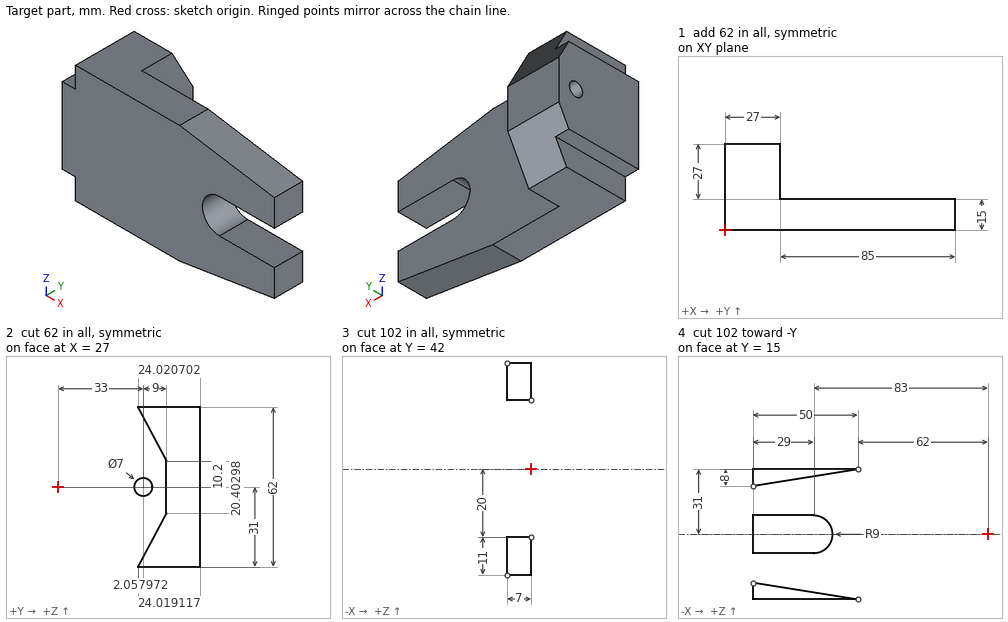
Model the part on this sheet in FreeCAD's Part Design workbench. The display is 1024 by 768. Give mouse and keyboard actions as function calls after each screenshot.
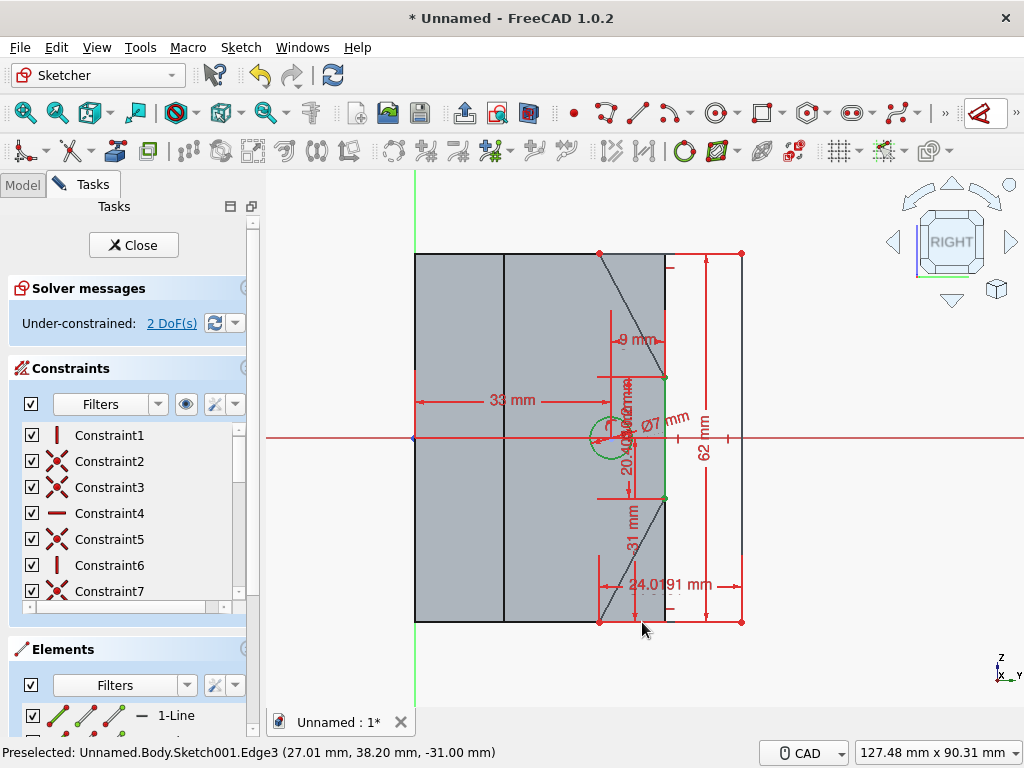
click(699, 254)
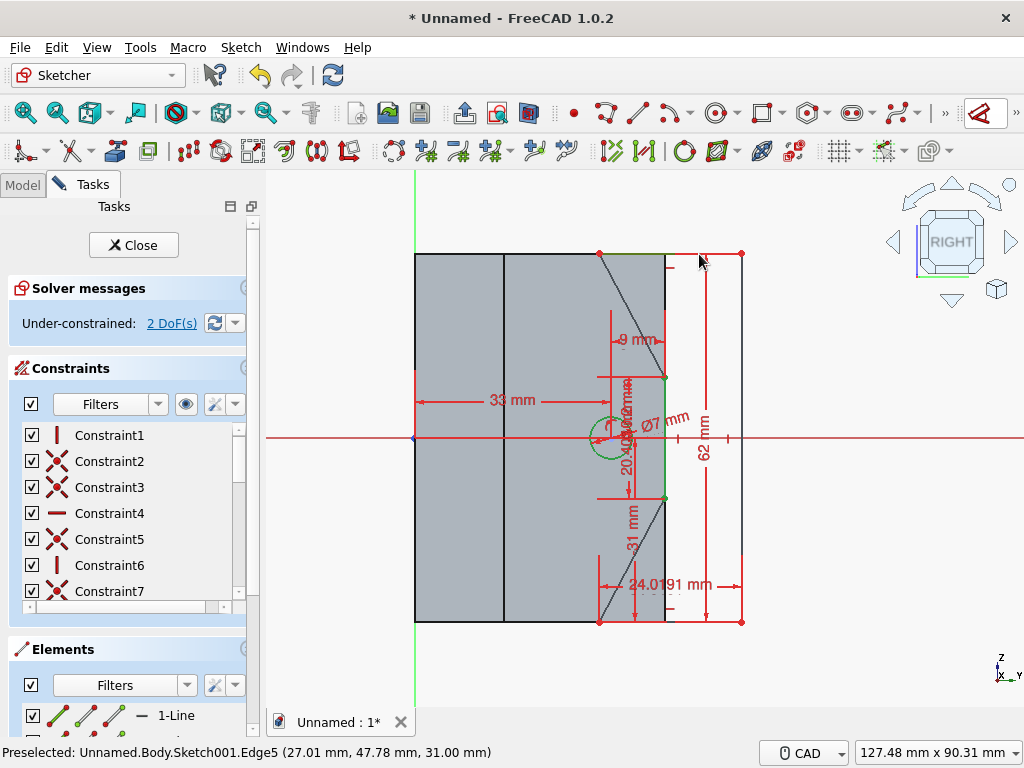
click(1002, 114)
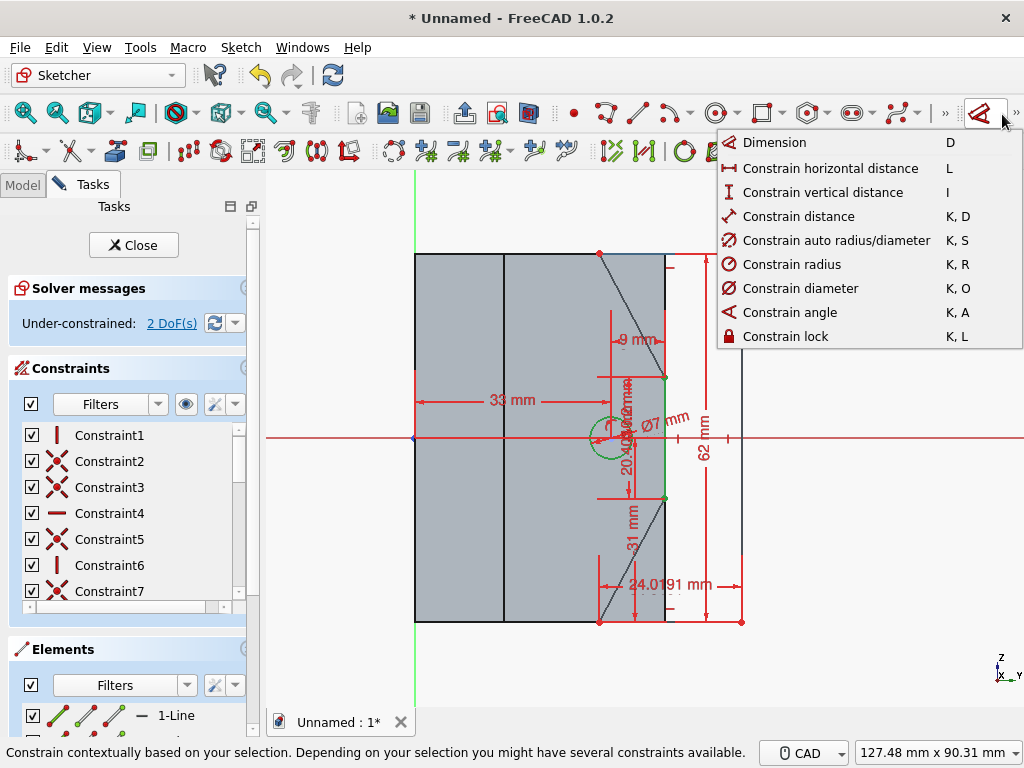
click(870, 168)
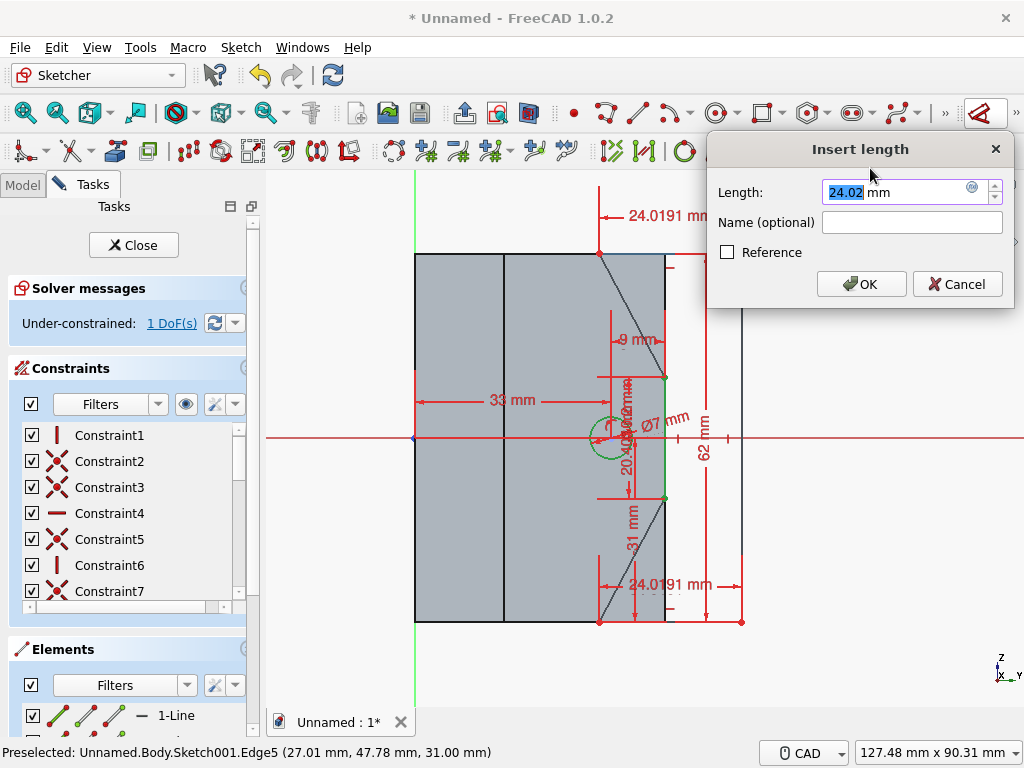
text(24.020702)
key(Return)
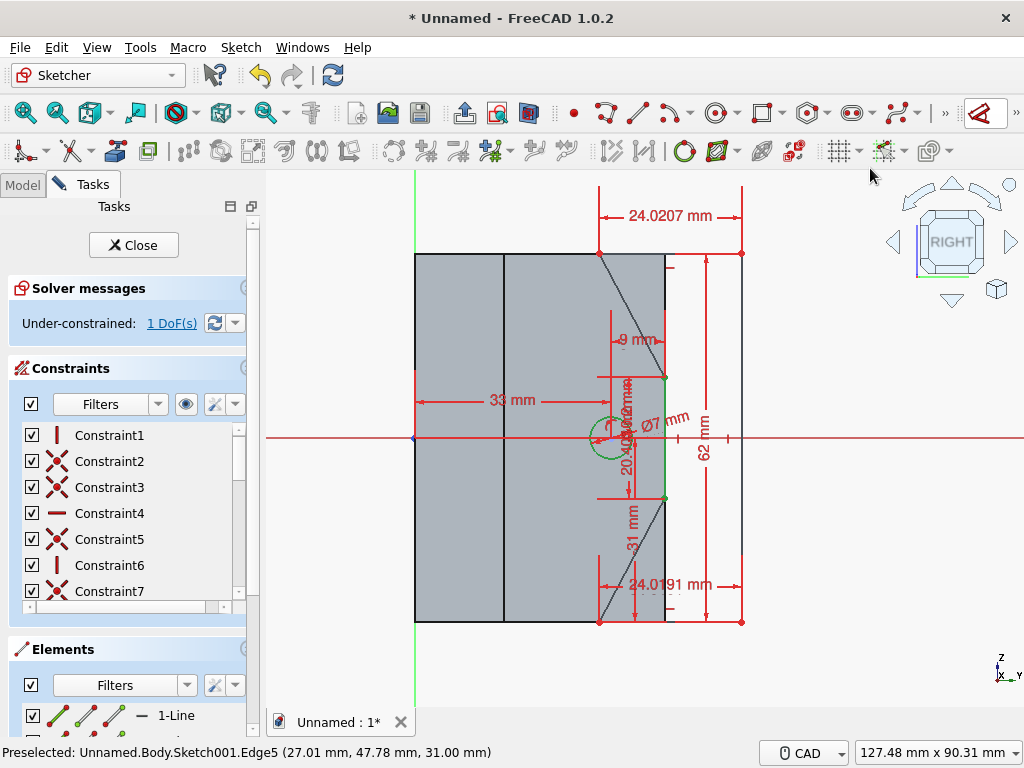
scroll(599, 622, up, 6)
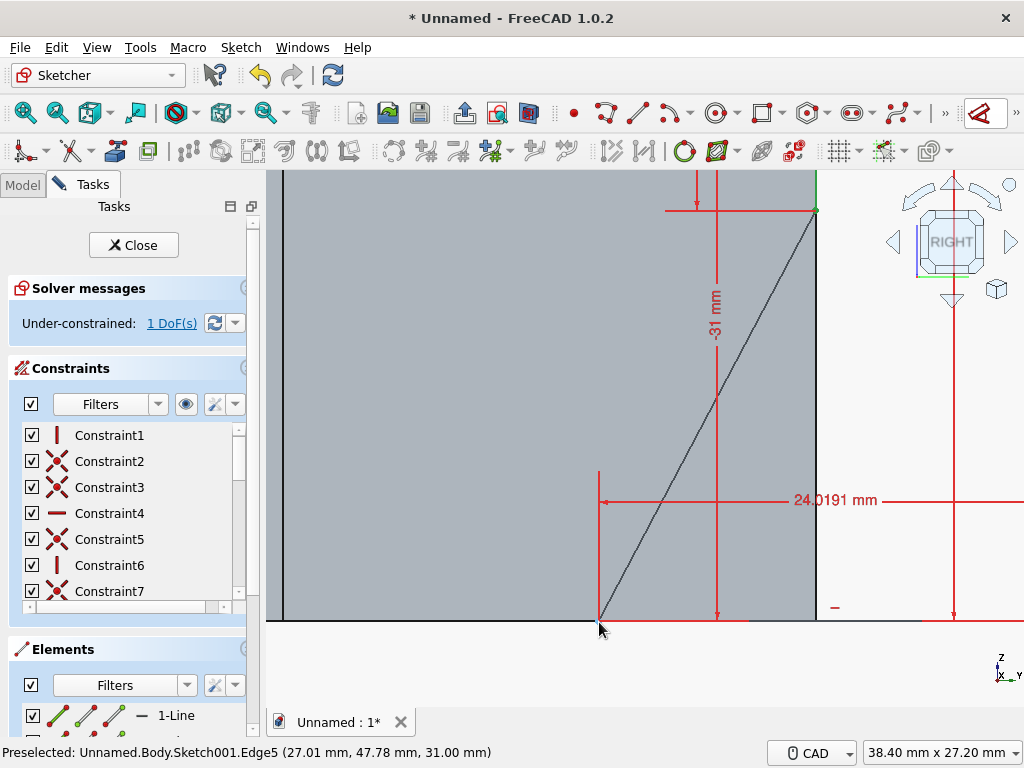
click(599, 621)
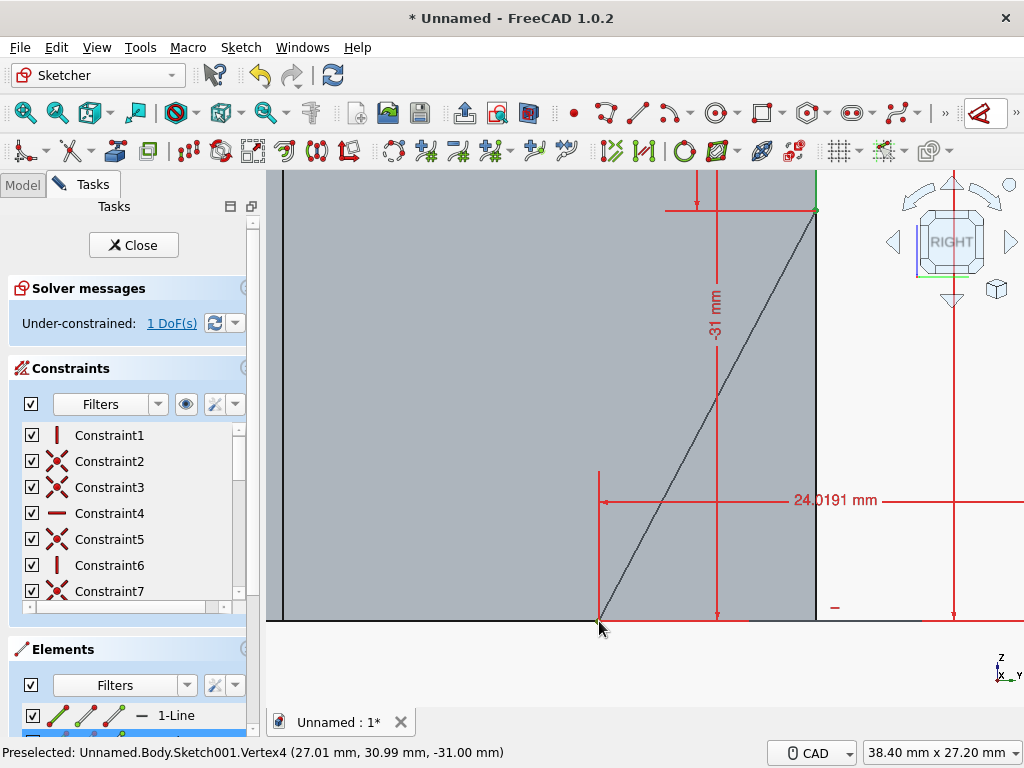
scroll(597, 624, down, 6)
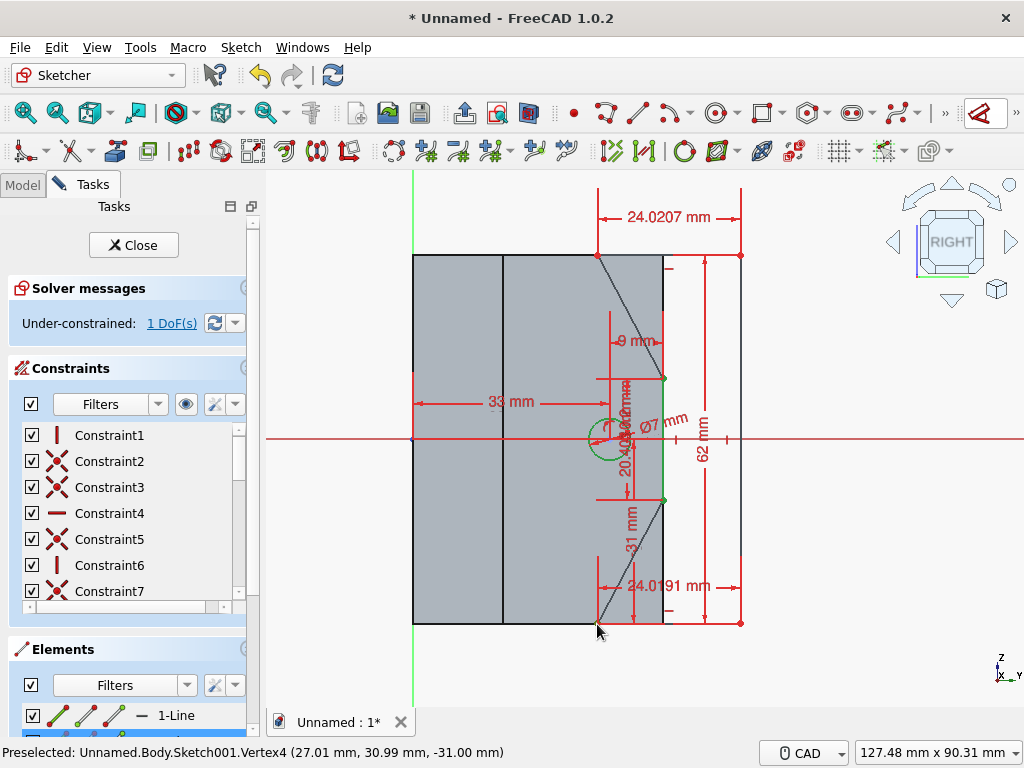
scroll(610, 439, up, 6)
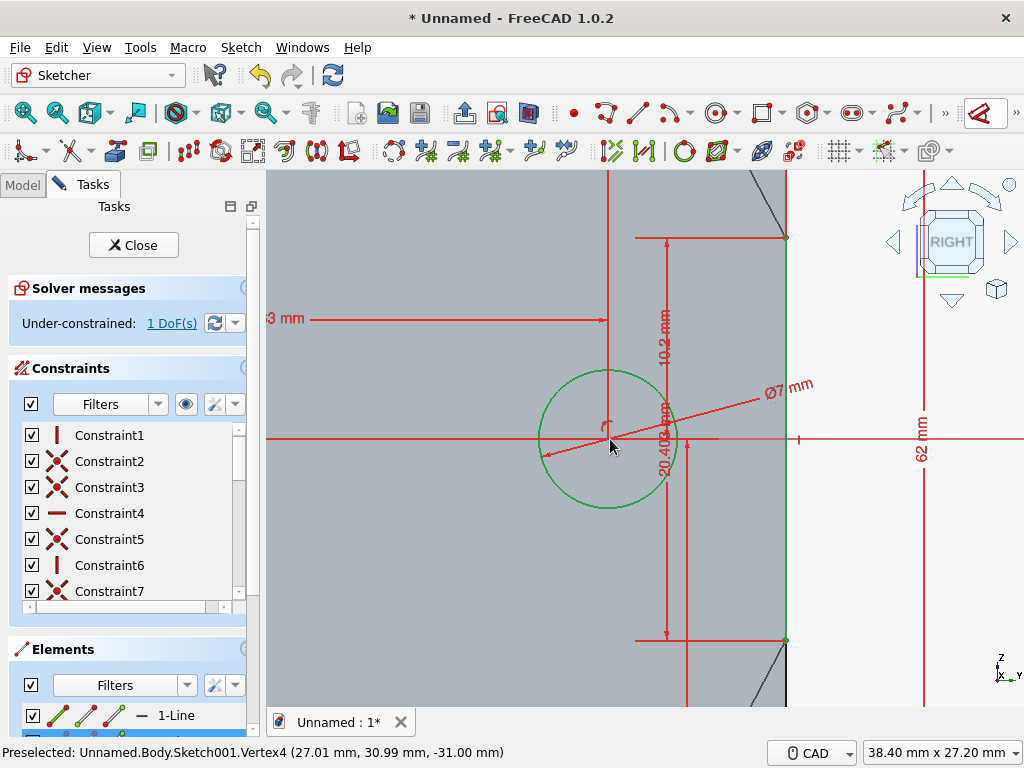
click(608, 439)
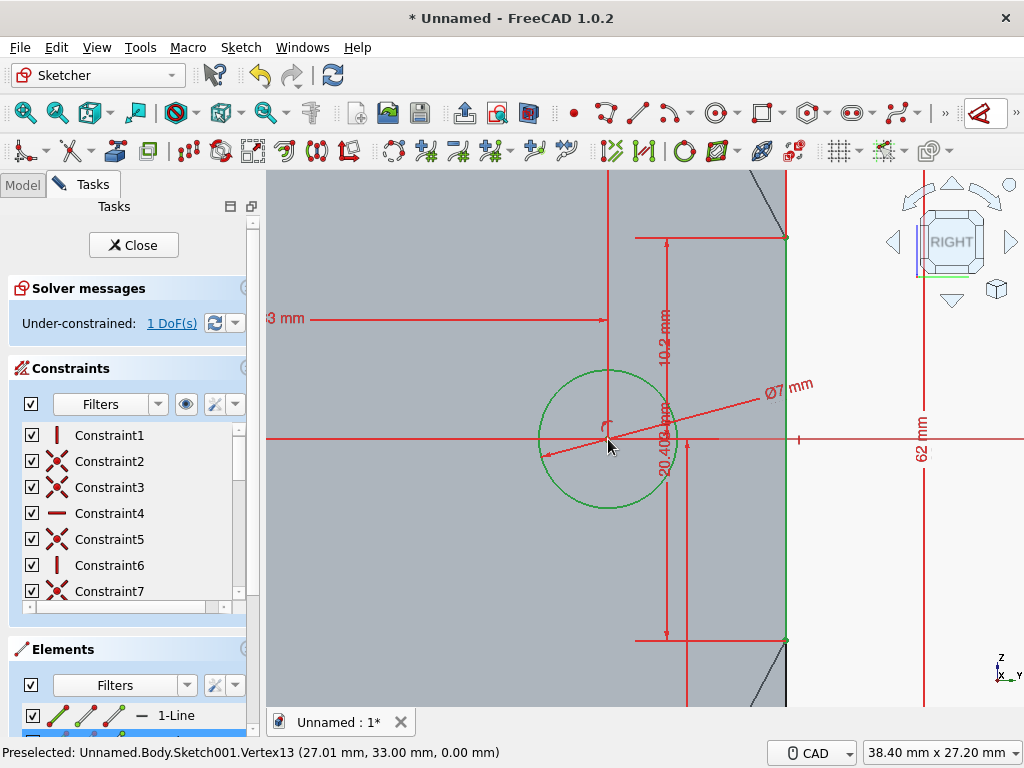
click(1002, 114)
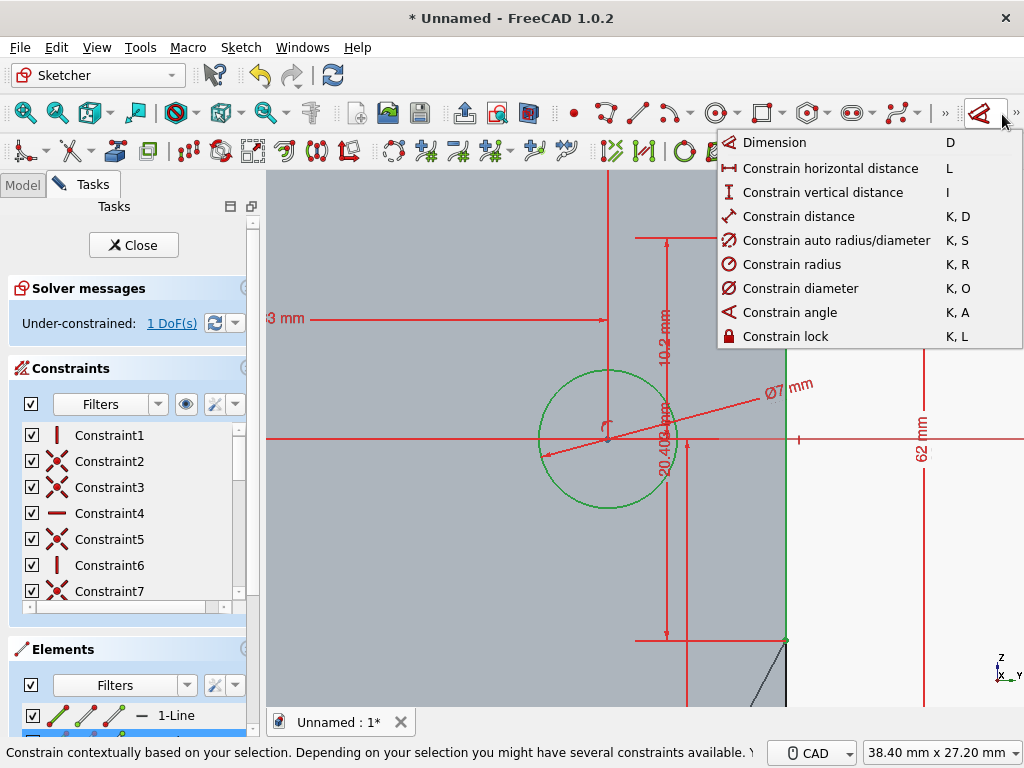
click(870, 168)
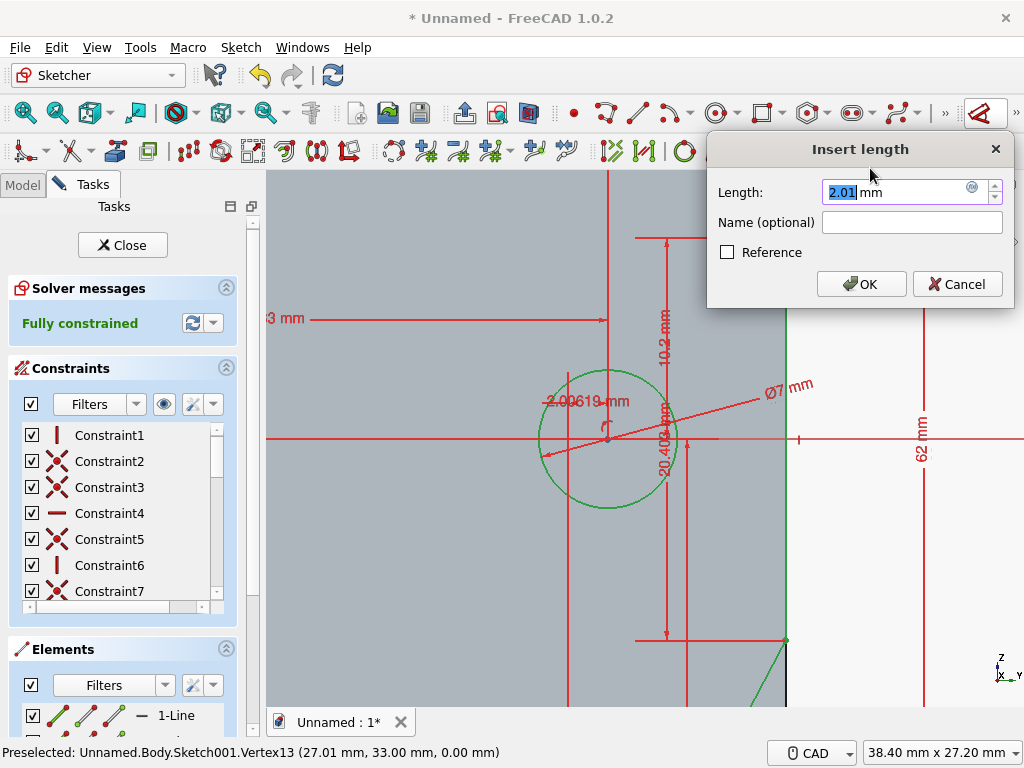
text(2.057972)
key(Return)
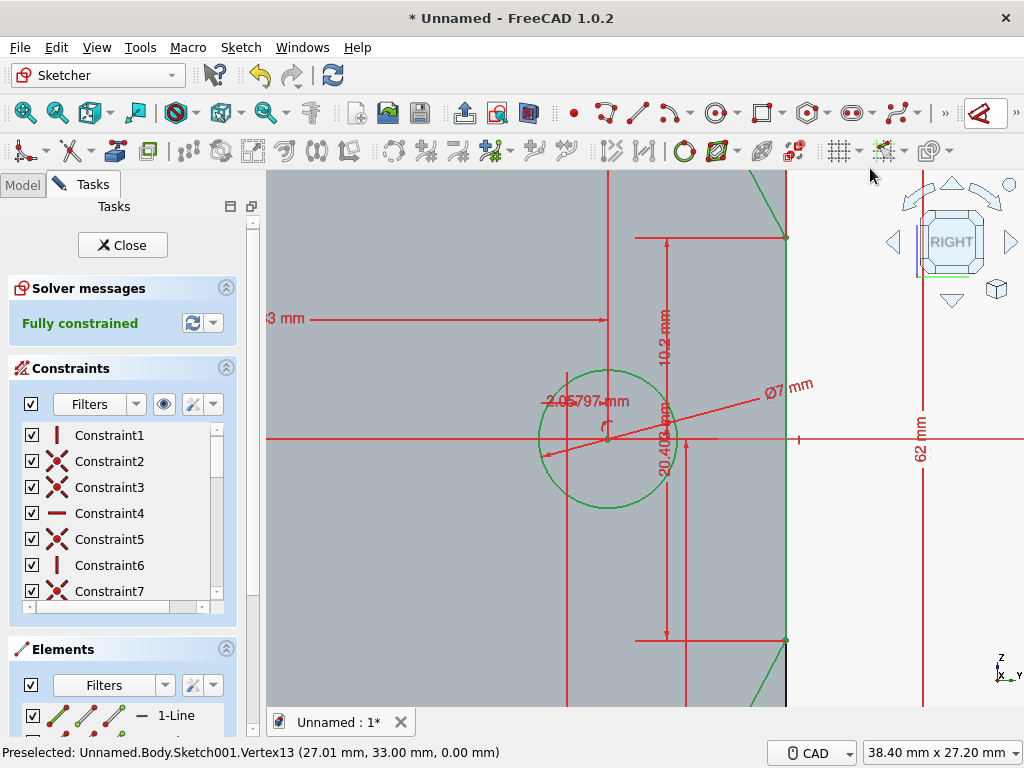
click(123, 245)